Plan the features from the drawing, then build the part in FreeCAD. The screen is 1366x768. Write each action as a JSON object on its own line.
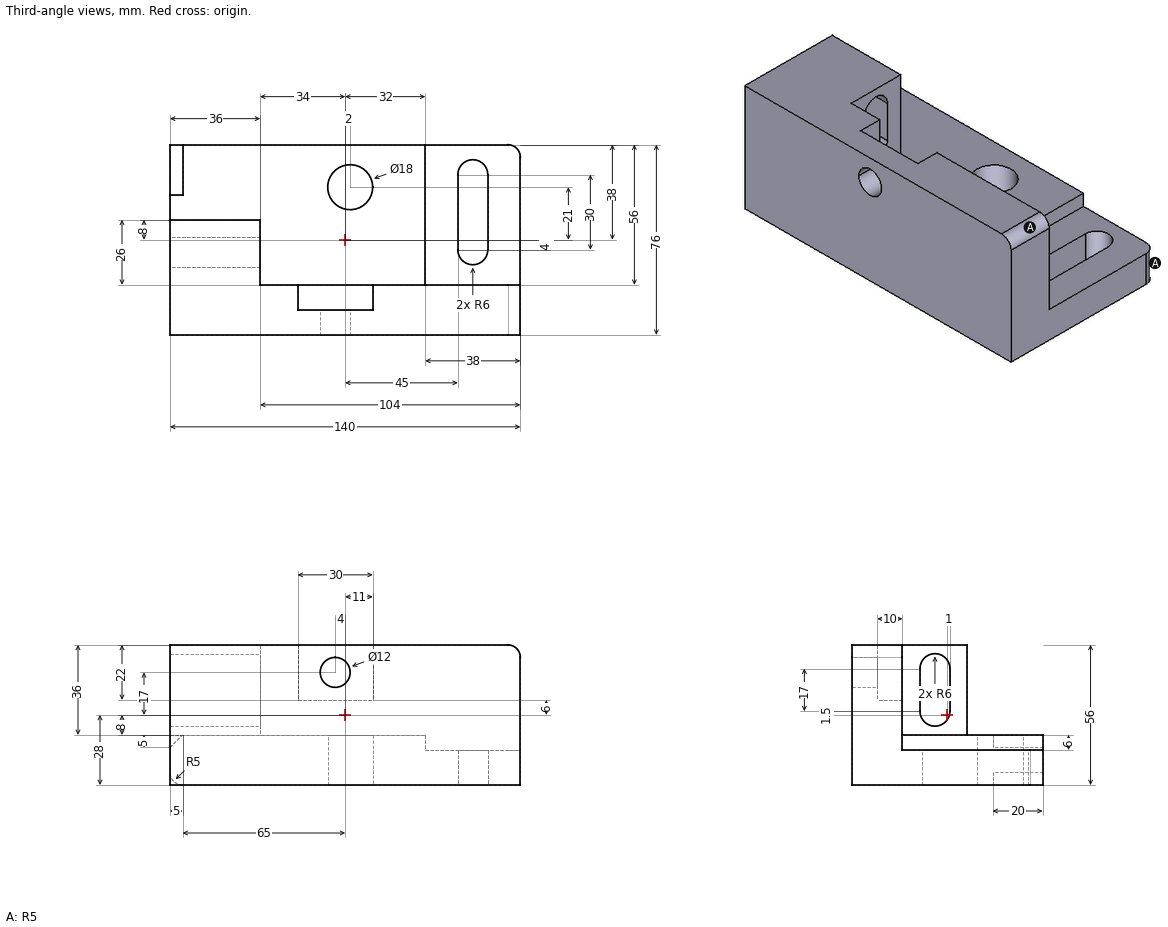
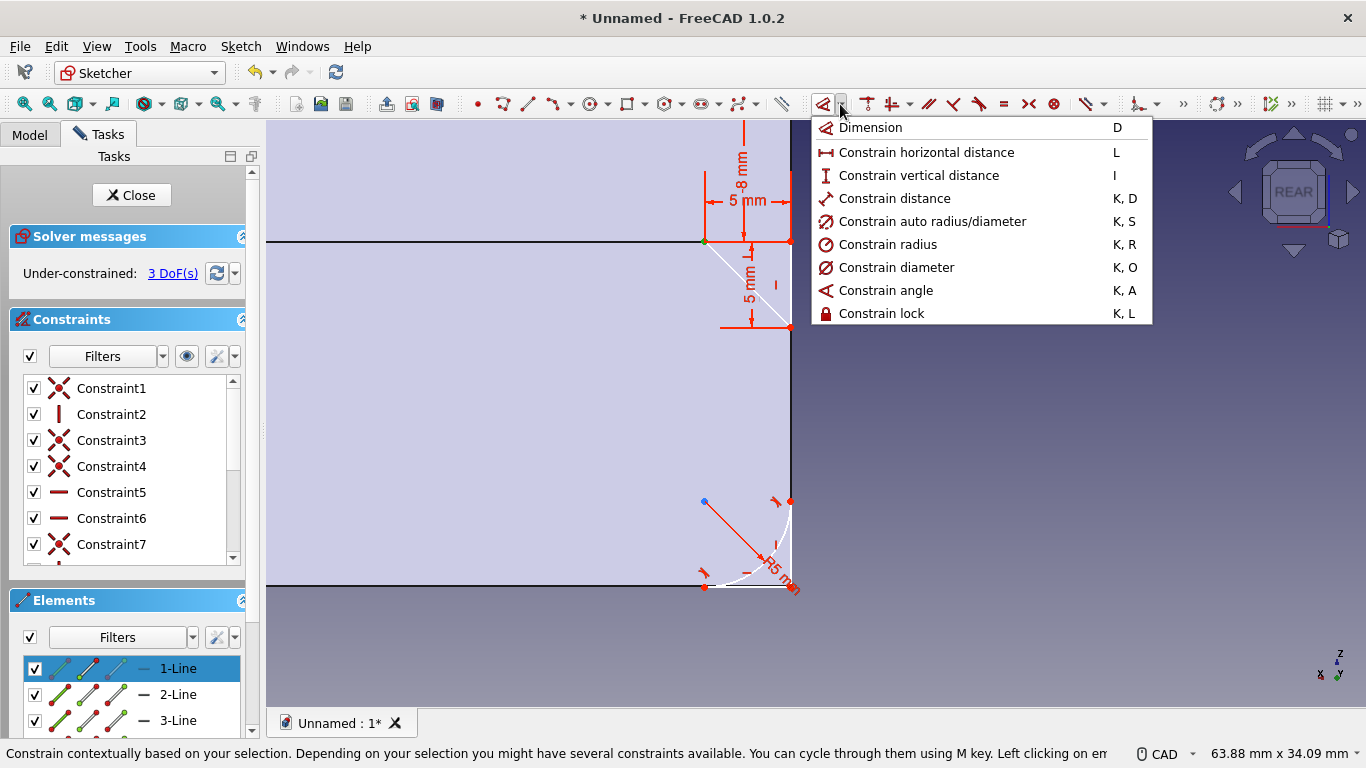
{"action": "left_click", "coordinate": [982, 152]}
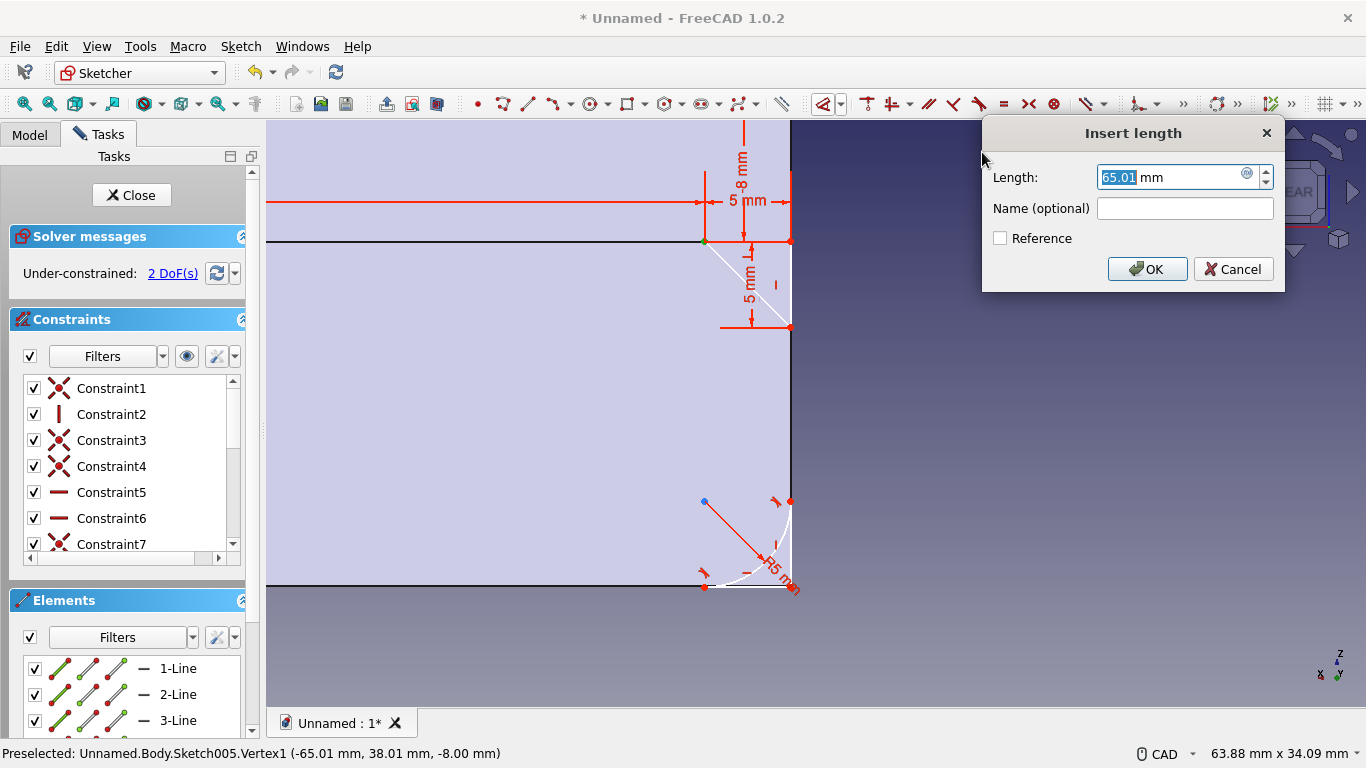
{"action": "type", "text": "65"}
{"action": "key", "text": "Return"}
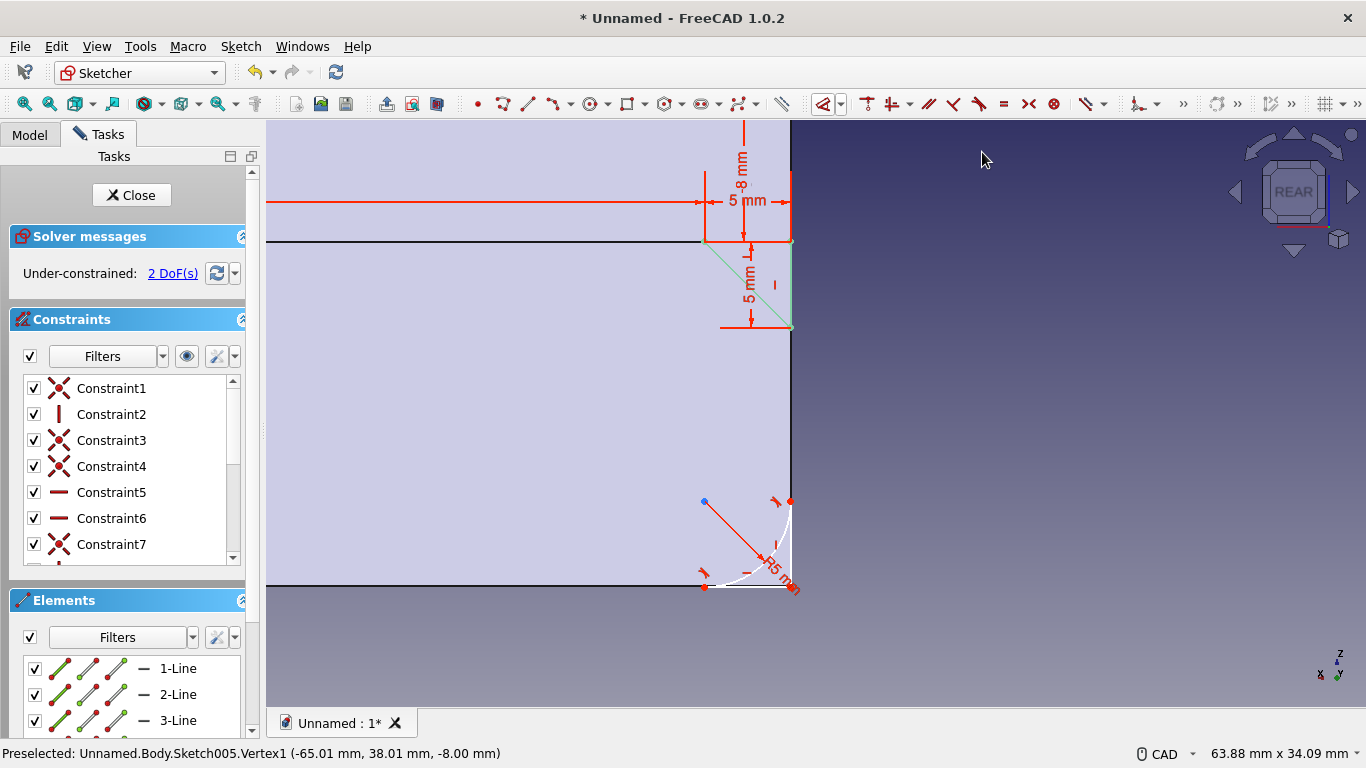
{"action": "left_click", "coordinate": [705, 587]}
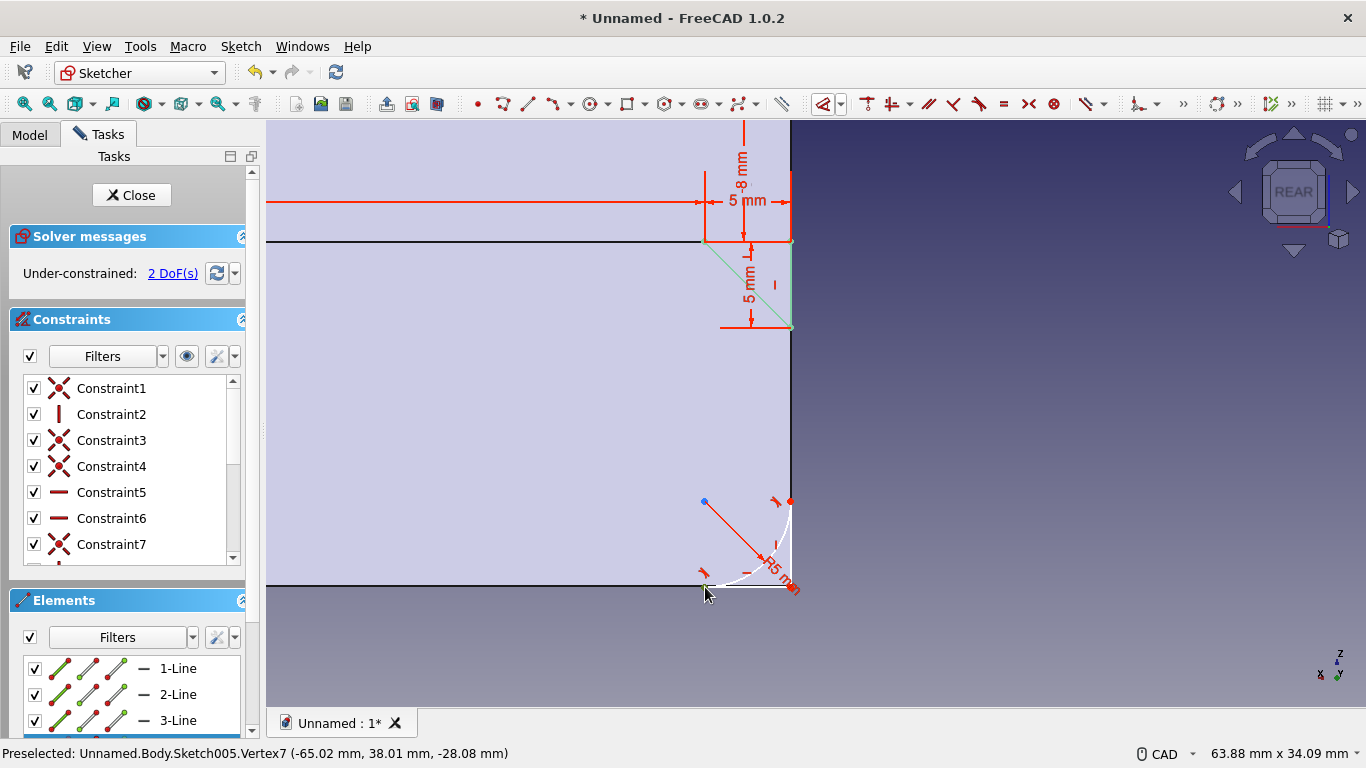
{"action": "left_click", "coordinate": [840, 104]}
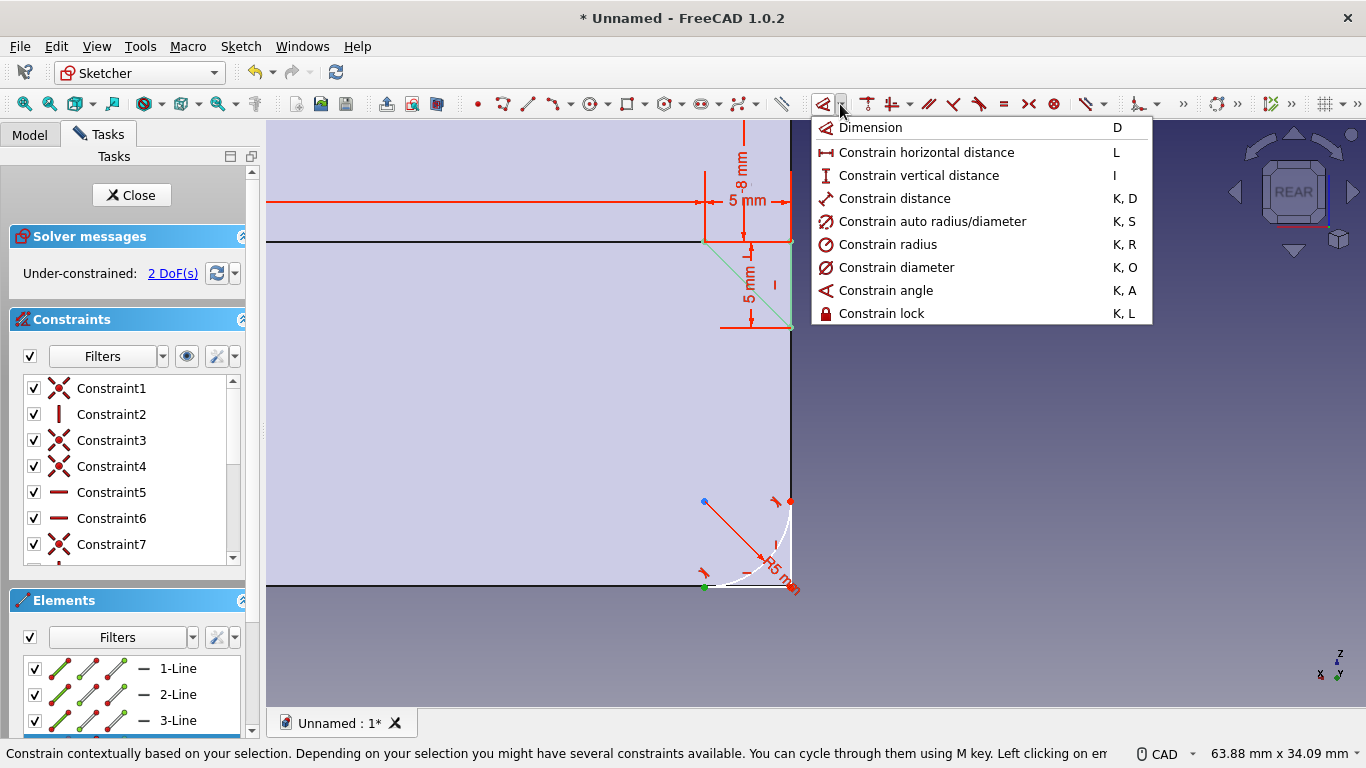
{"action": "left_click", "coordinate": [982, 152]}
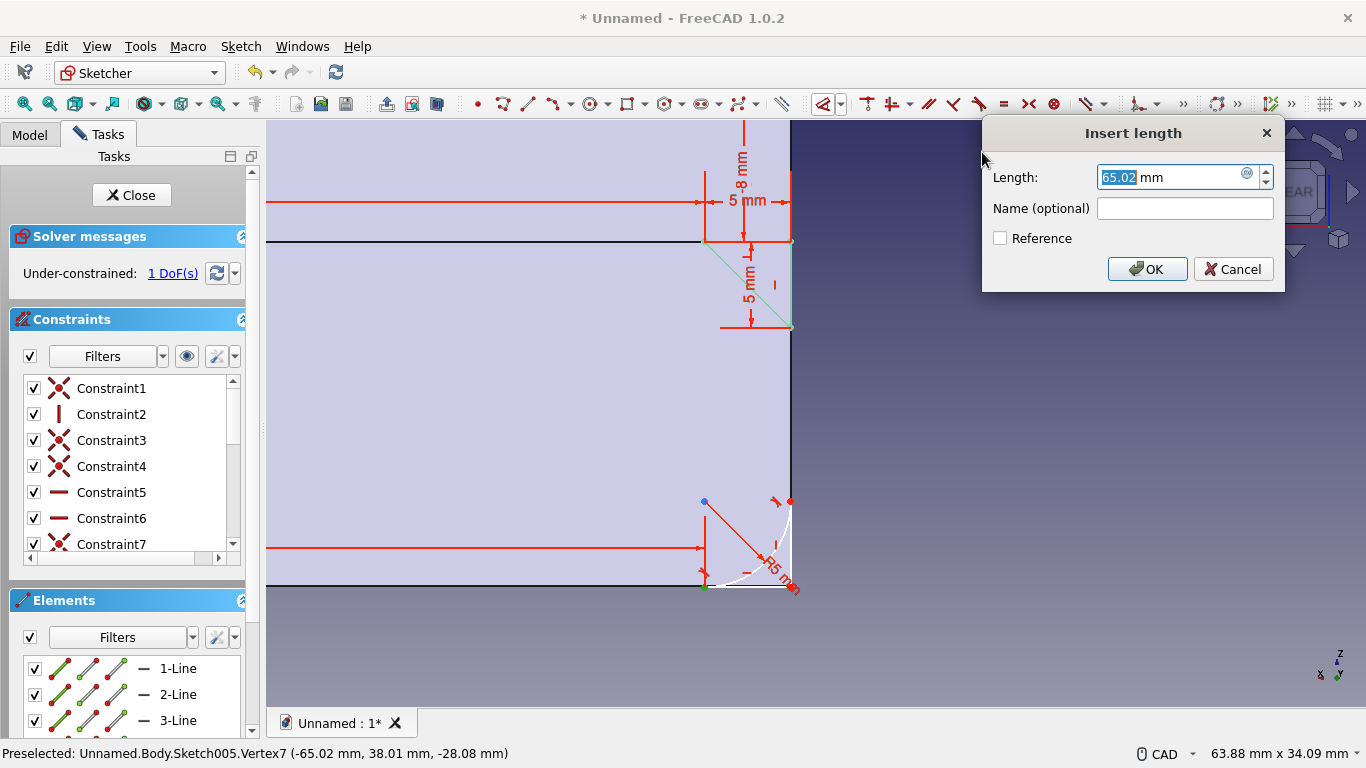
{"action": "type", "text": "65"}
{"action": "key", "text": "Return"}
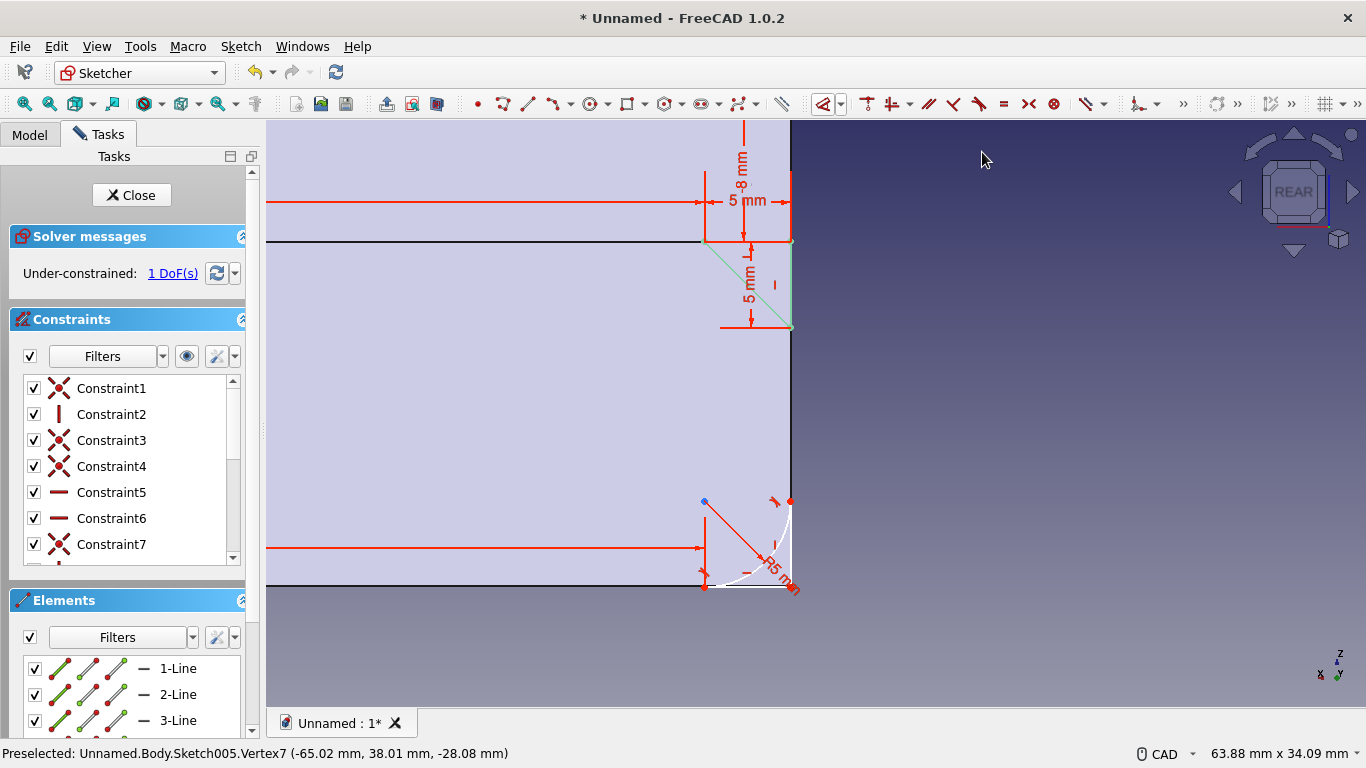
{"action": "left_click", "coordinate": [705, 587]}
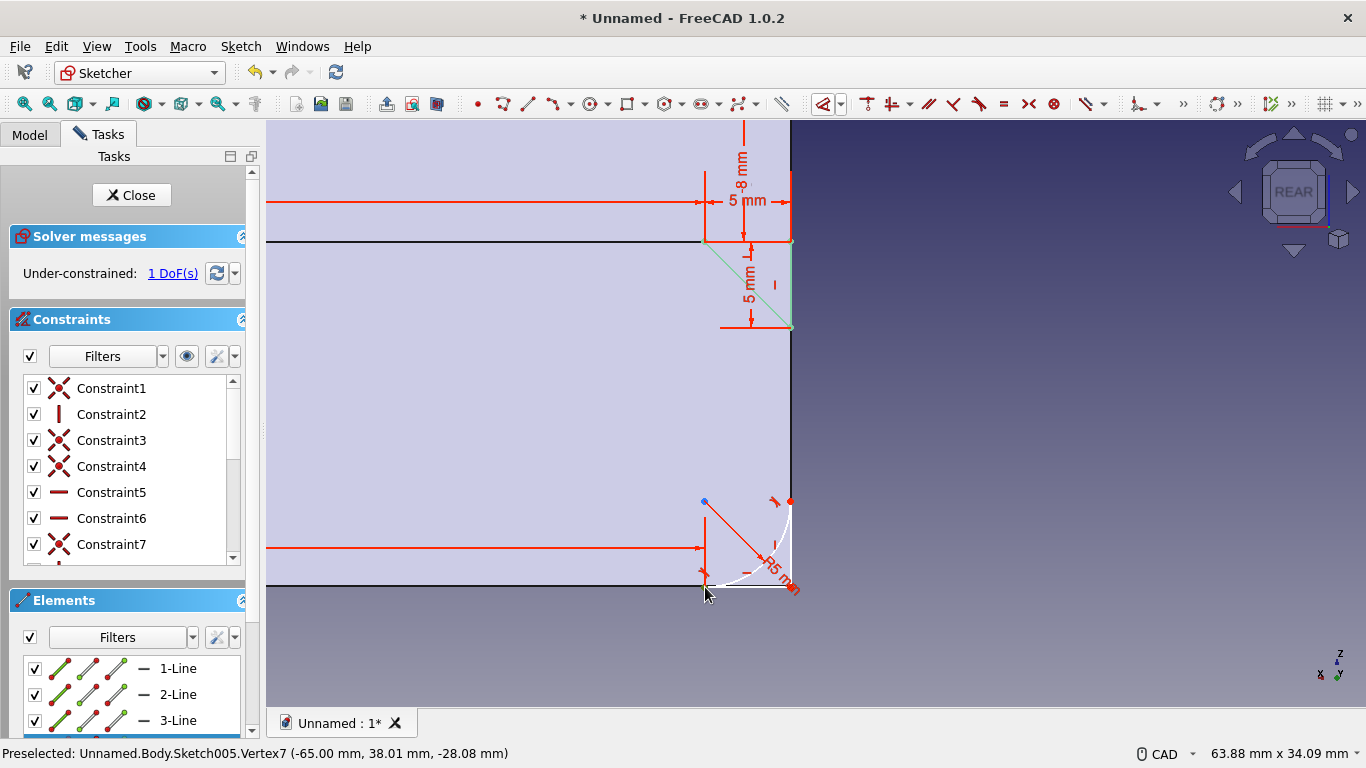
{"action": "left_click", "coordinate": [840, 104]}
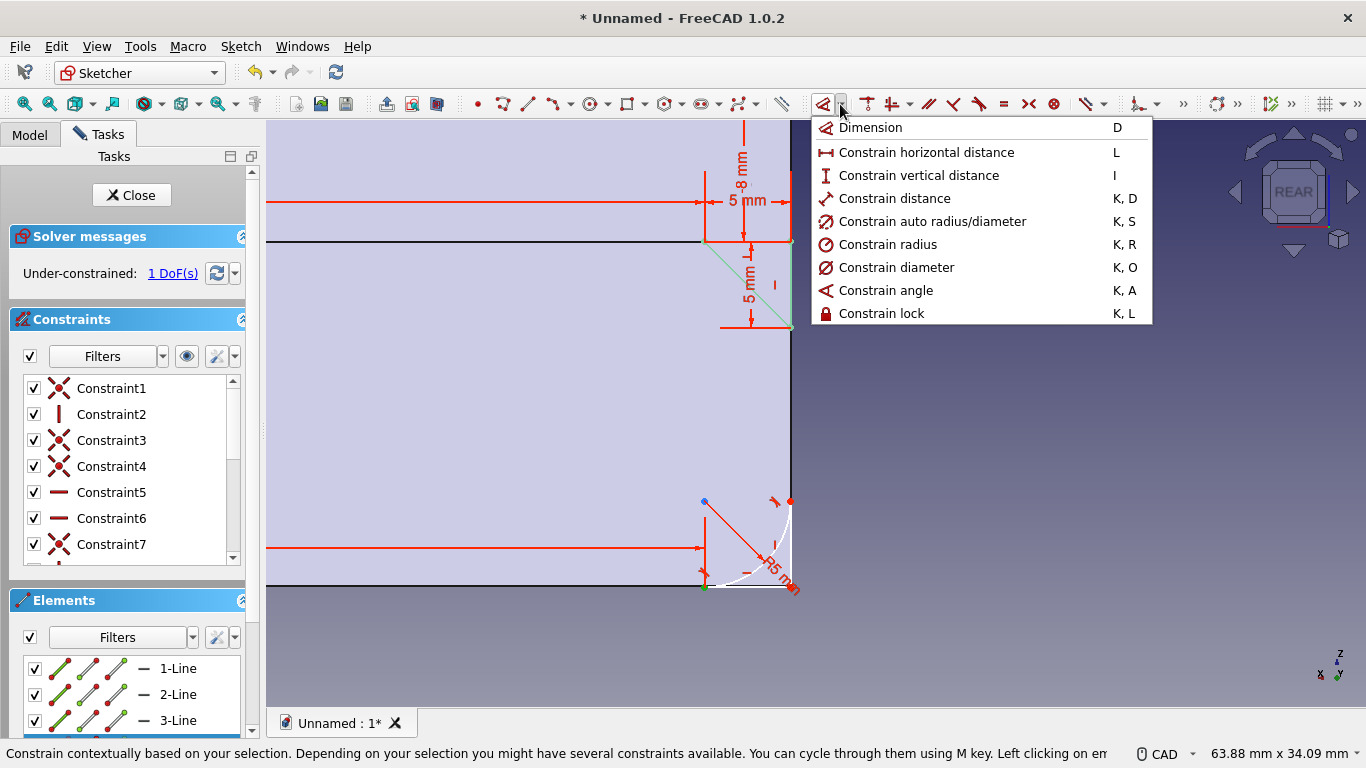
{"action": "left_click", "coordinate": [982, 176]}